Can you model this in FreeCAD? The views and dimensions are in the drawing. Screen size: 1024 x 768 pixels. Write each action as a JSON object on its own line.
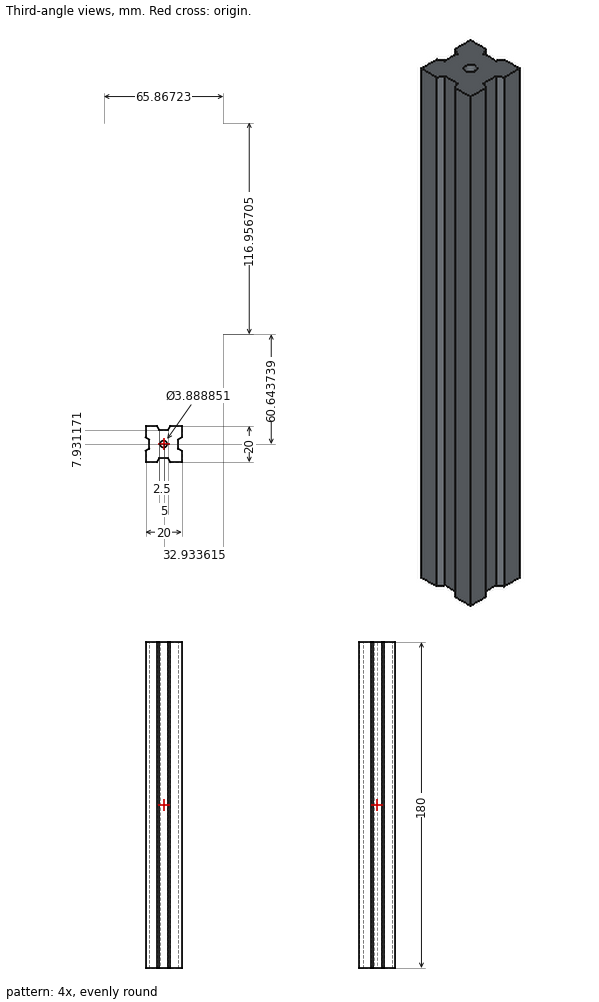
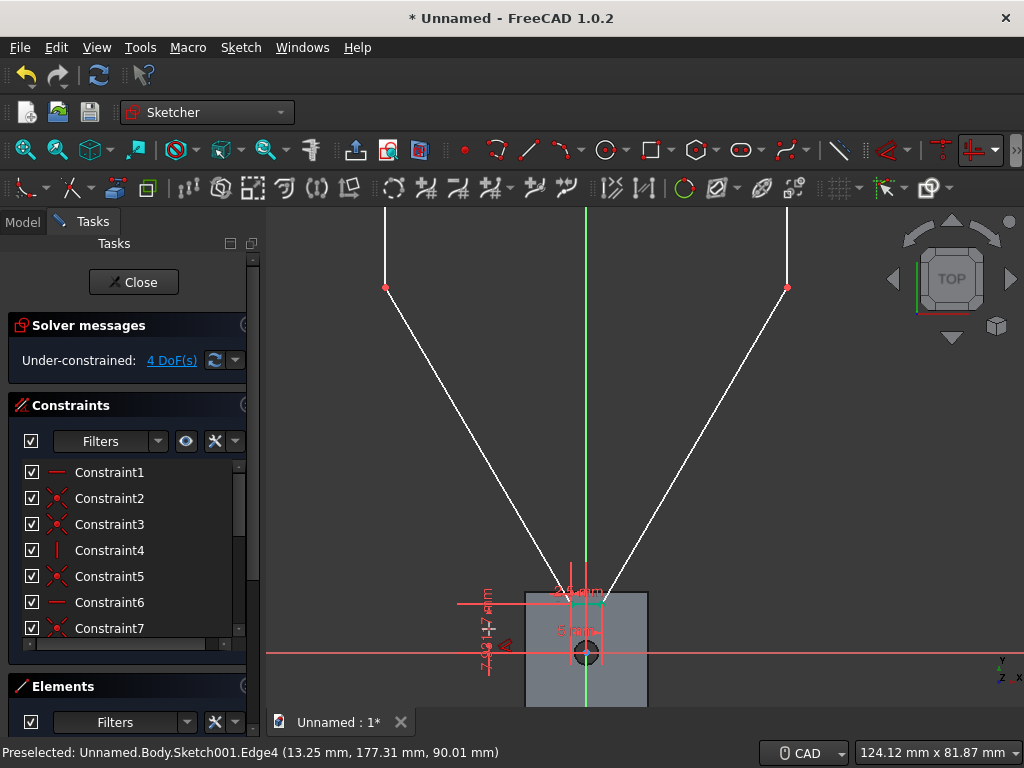
{"action": "scroll", "coordinate": [572, 606], "scroll_direction": "down", "scroll_amount": 6}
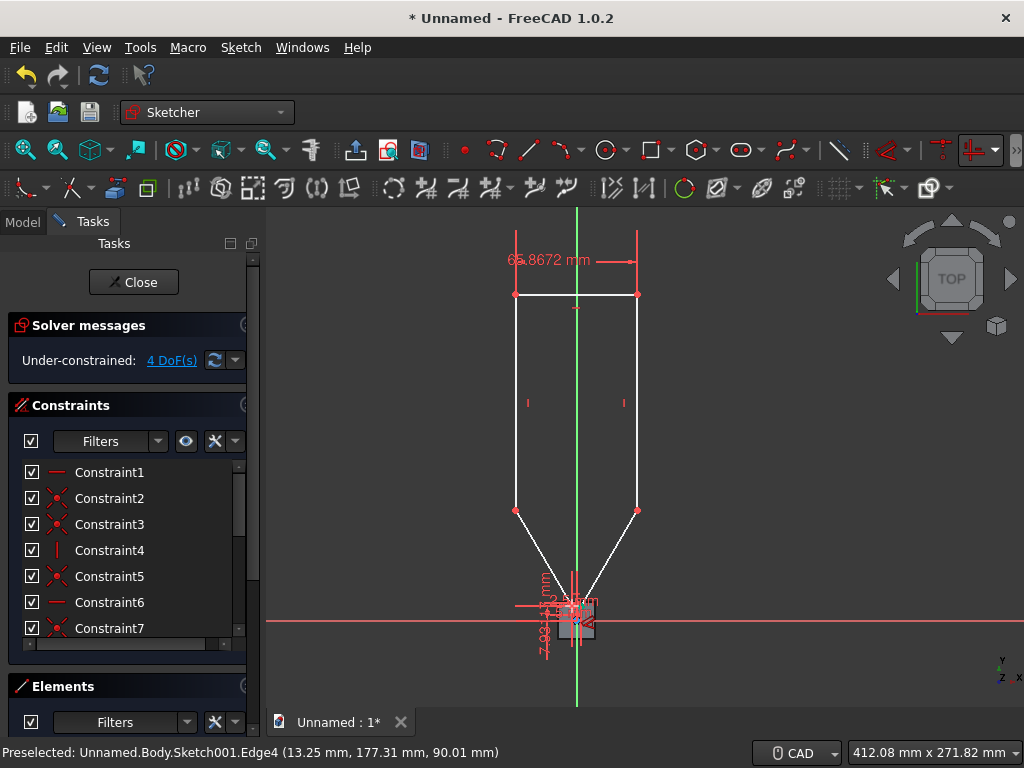
{"action": "left_click", "coordinate": [637, 446]}
{"action": "left_click", "coordinate": [671, 403]}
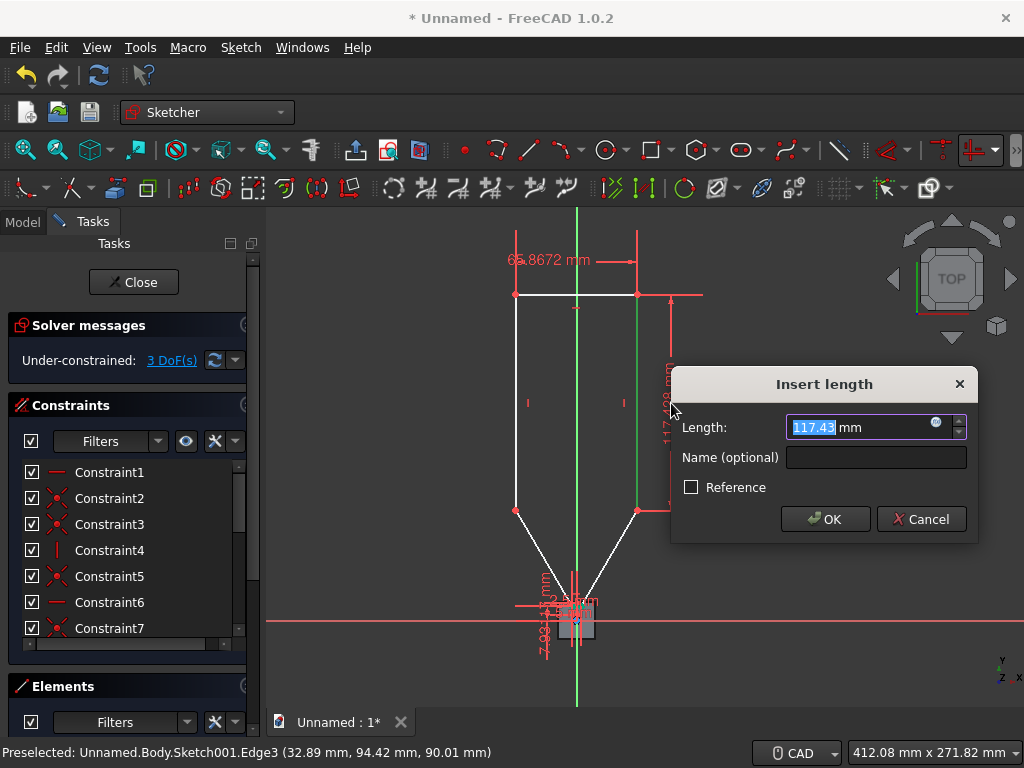
{"action": "type", "text": "116.956705"}
{"action": "key", "text": "Return"}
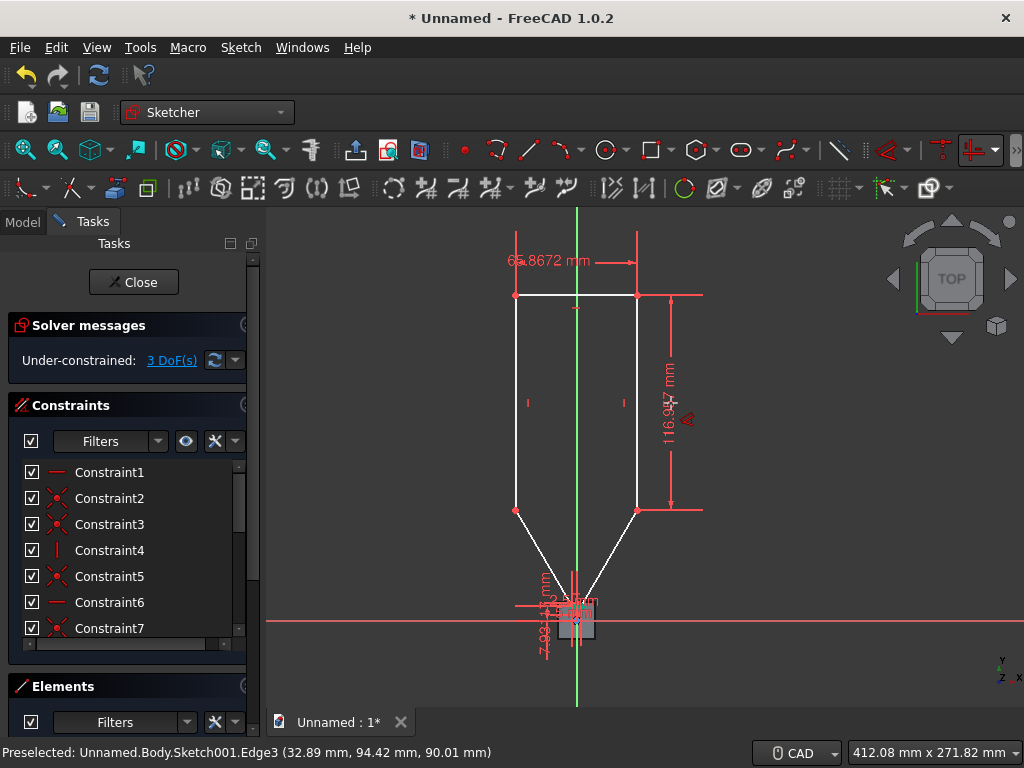
{"action": "left_click", "coordinate": [516, 360]}
{"action": "left_click", "coordinate": [482, 403]}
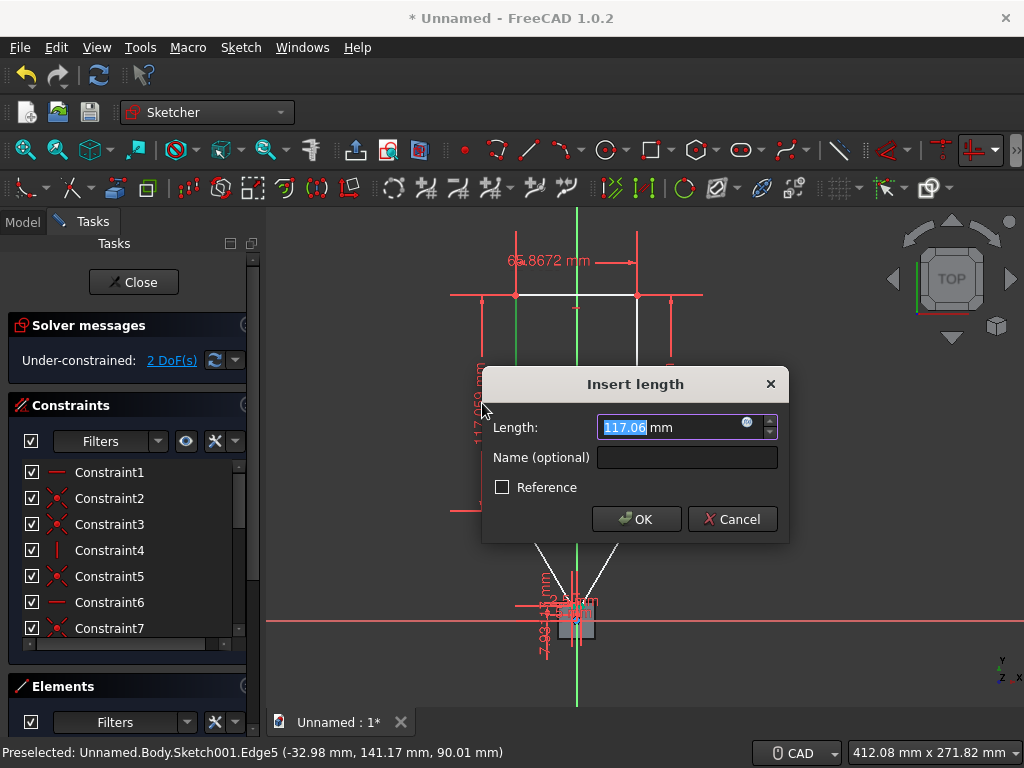
{"action": "type", "text": "116.956705"}
{"action": "key", "text": "Return"}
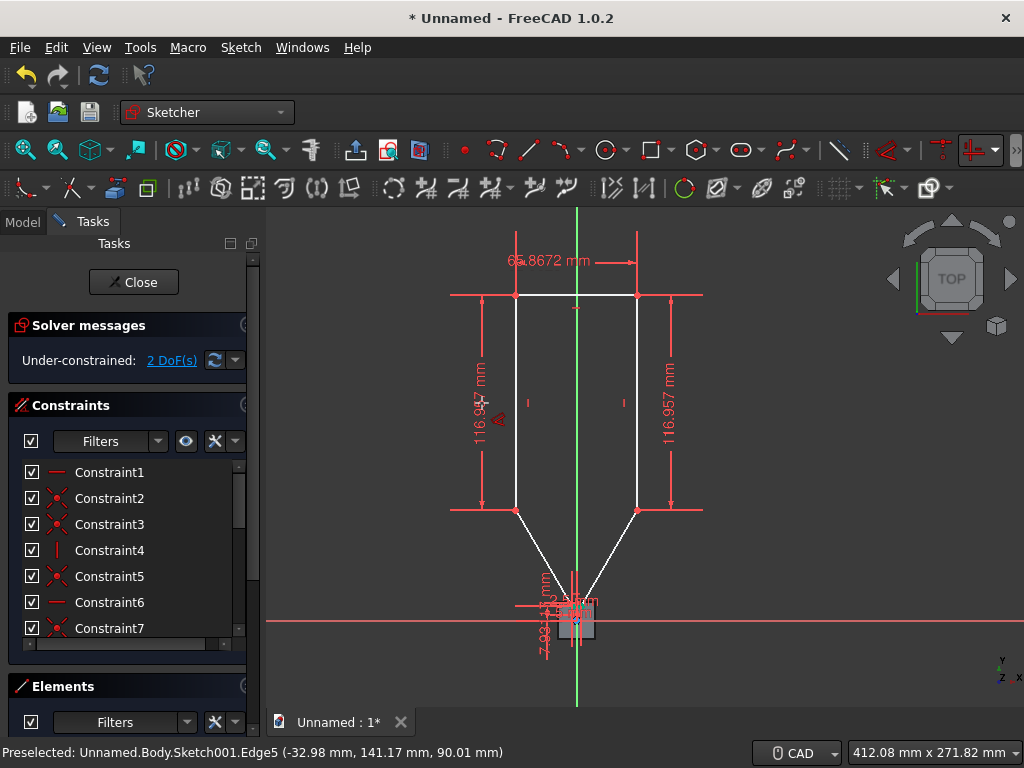
{"action": "left_click", "coordinate": [637, 510]}
{"action": "left_click", "coordinate": [607, 655]}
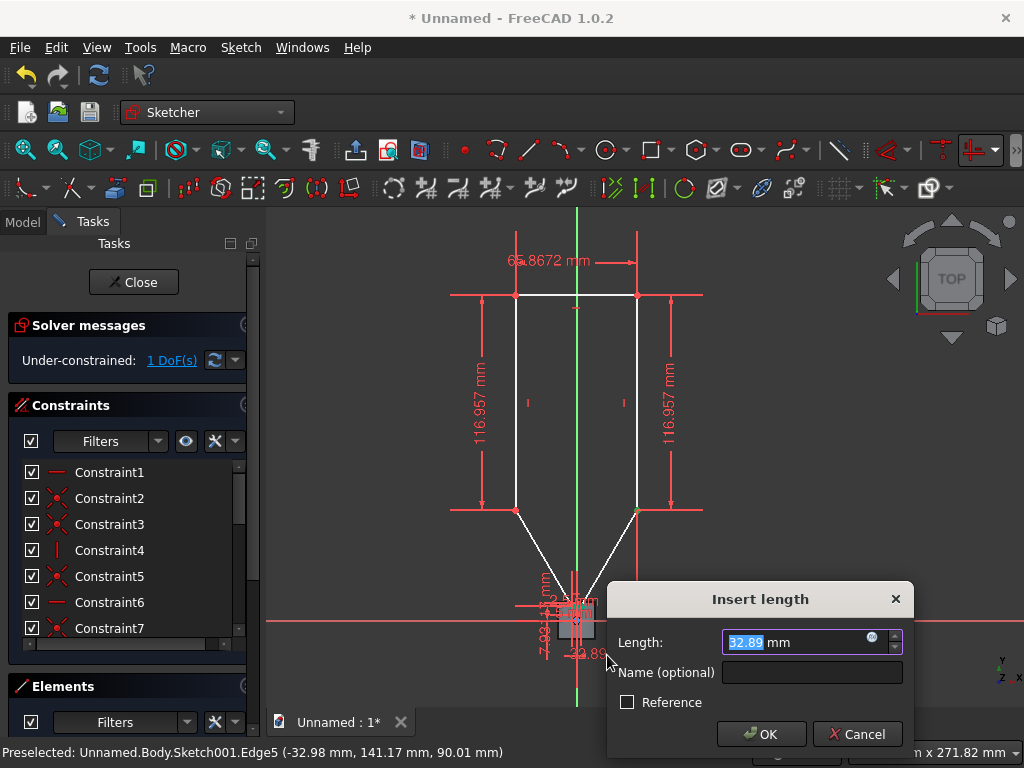
{"action": "type", "text": "32.933615"}
{"action": "key", "text": "Return"}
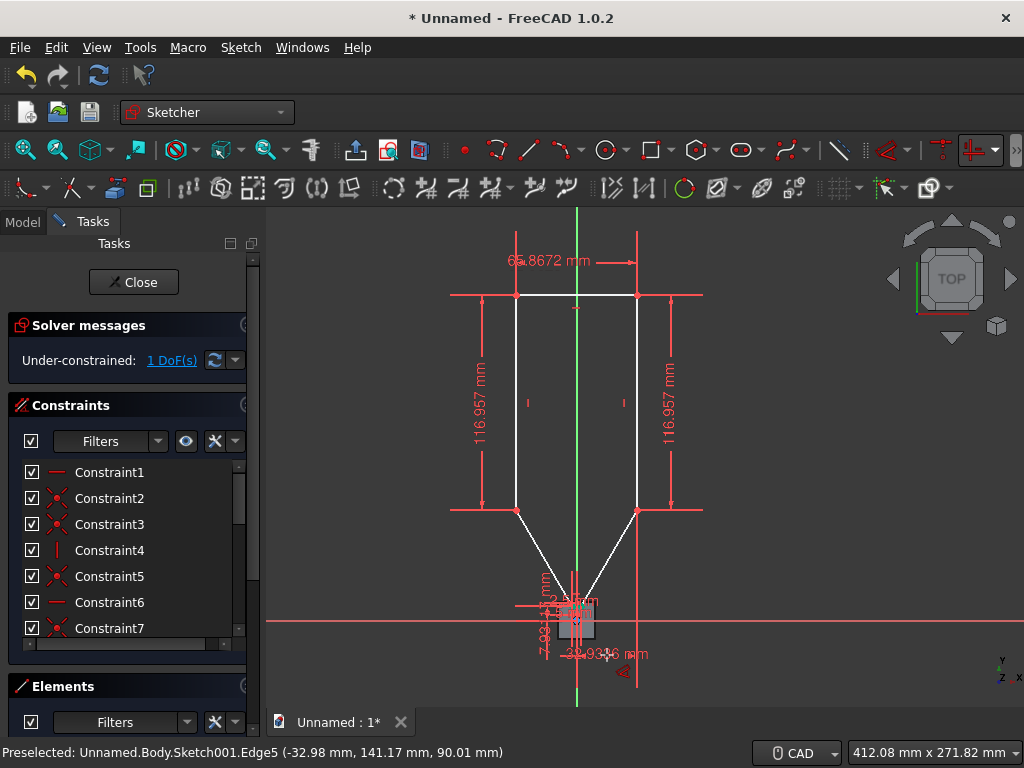
{"action": "left_click", "coordinate": [637, 510]}
{"action": "left_click", "coordinate": [671, 566]}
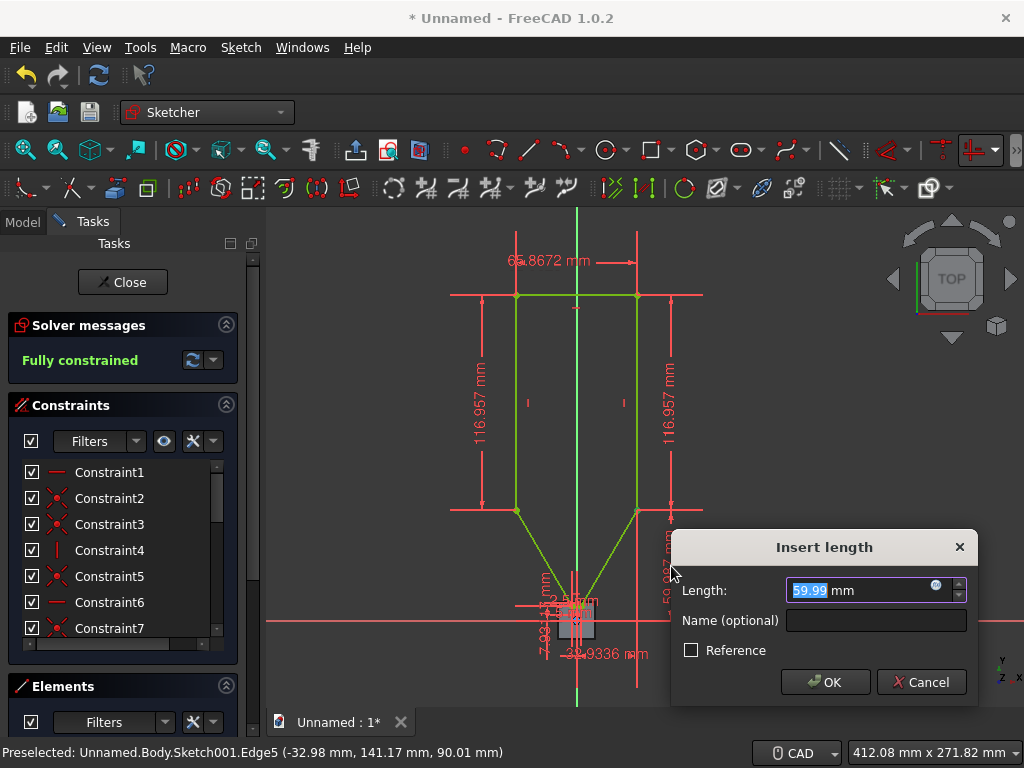
{"action": "type", "text": "60.643739"}
{"action": "key", "text": "Return"}
{"action": "key", "text": "Escape"}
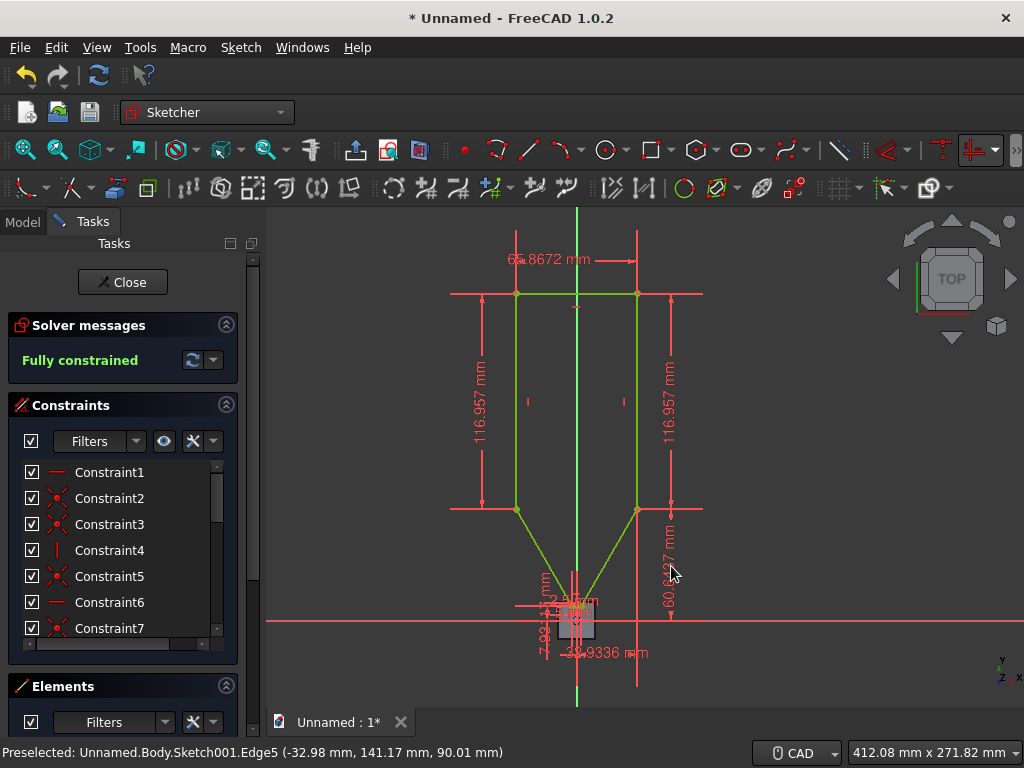
{"action": "left_click", "coordinate": [123, 282]}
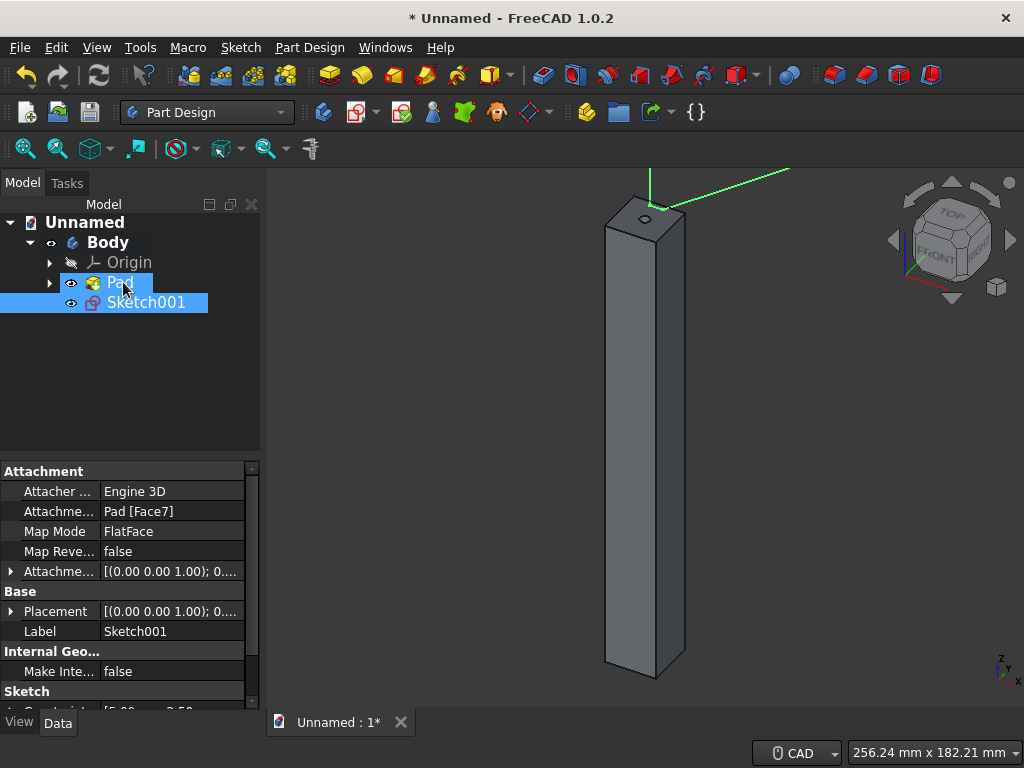
{"action": "left_click", "coordinate": [544, 76]}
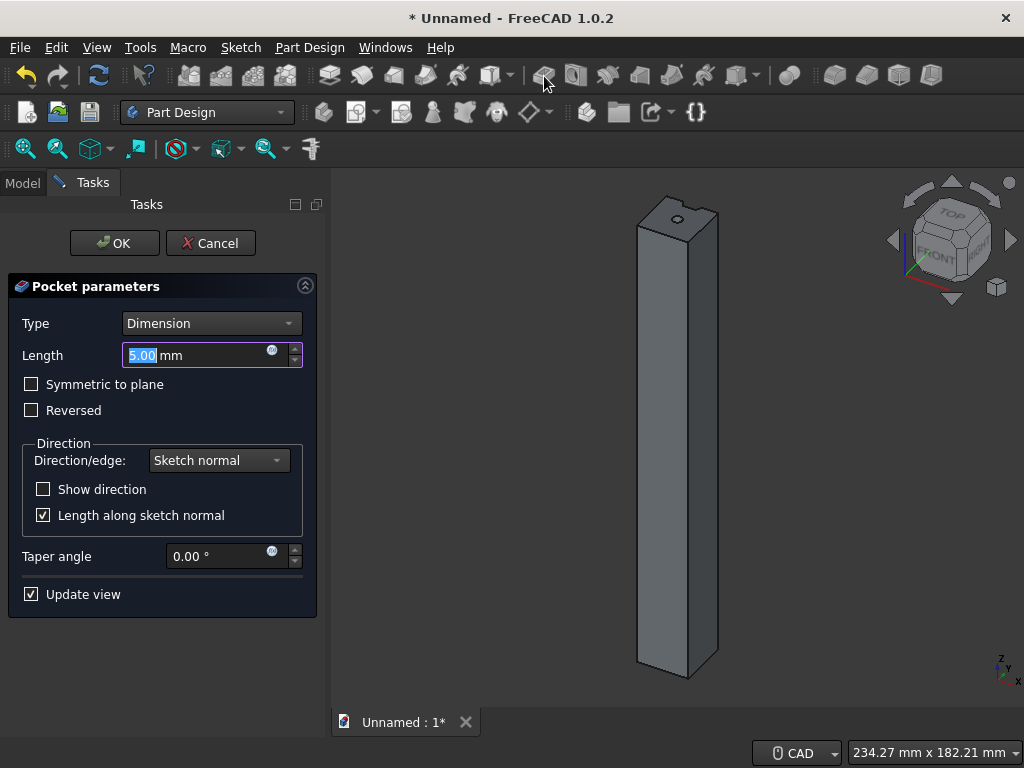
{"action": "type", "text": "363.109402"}
{"action": "key", "text": "Tab"}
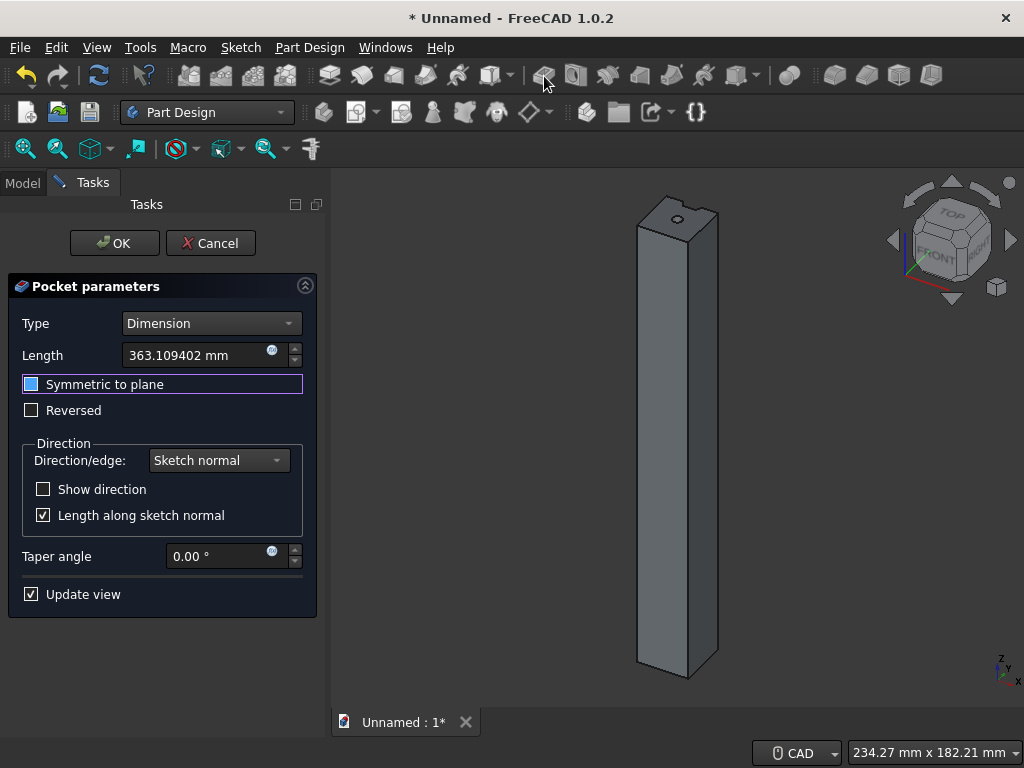
{"action": "left_click", "coordinate": [30, 384]}